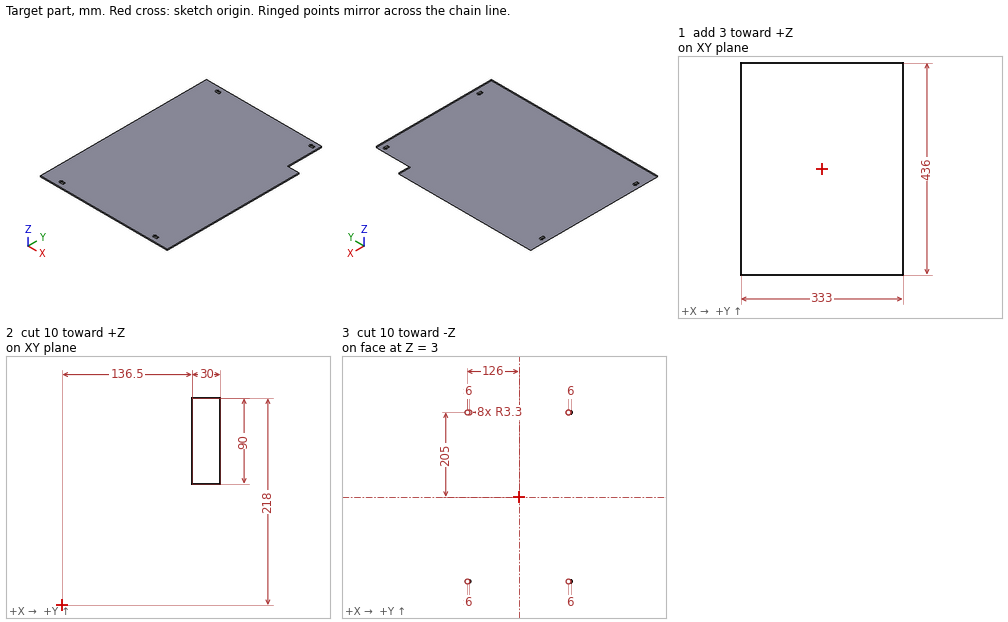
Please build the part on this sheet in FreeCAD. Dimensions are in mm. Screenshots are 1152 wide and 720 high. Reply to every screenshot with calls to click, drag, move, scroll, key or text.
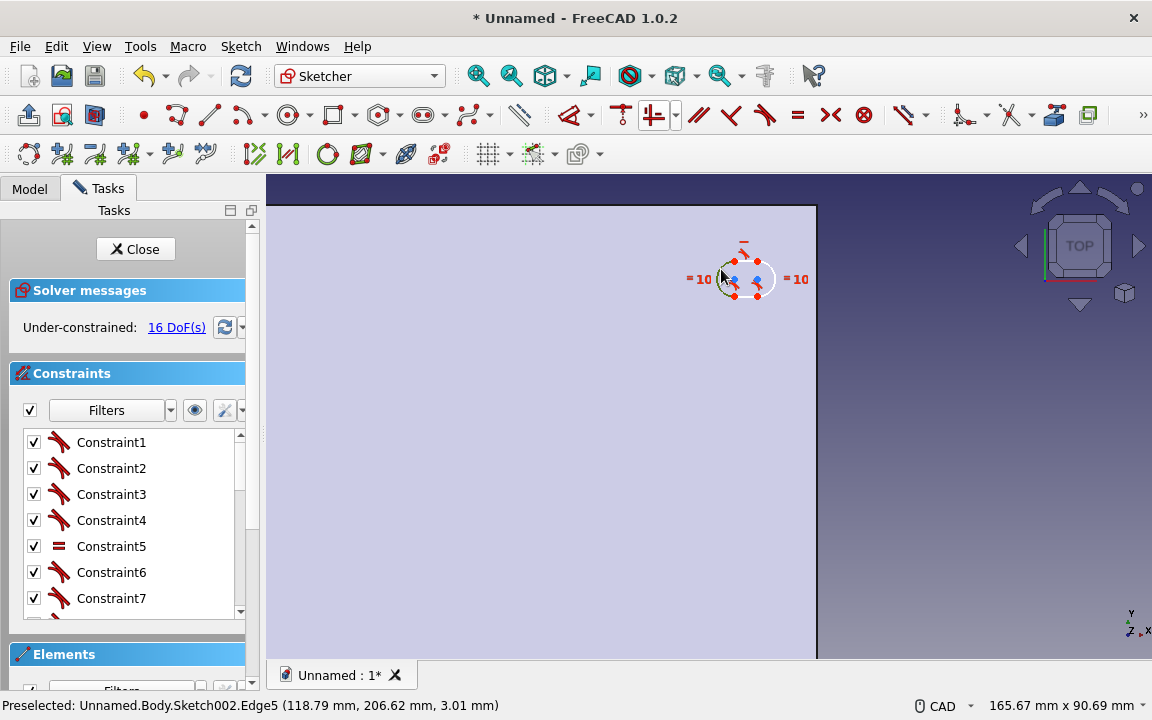
scroll(727, 267, down, 10)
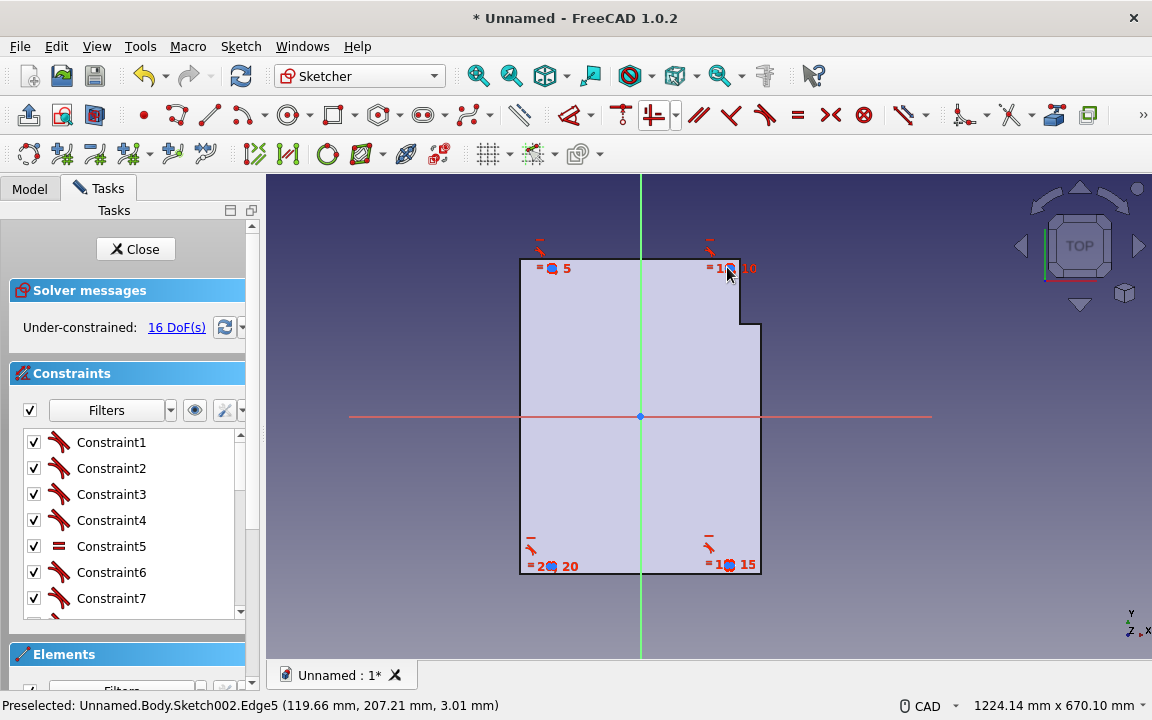
scroll(726, 564, up, 9)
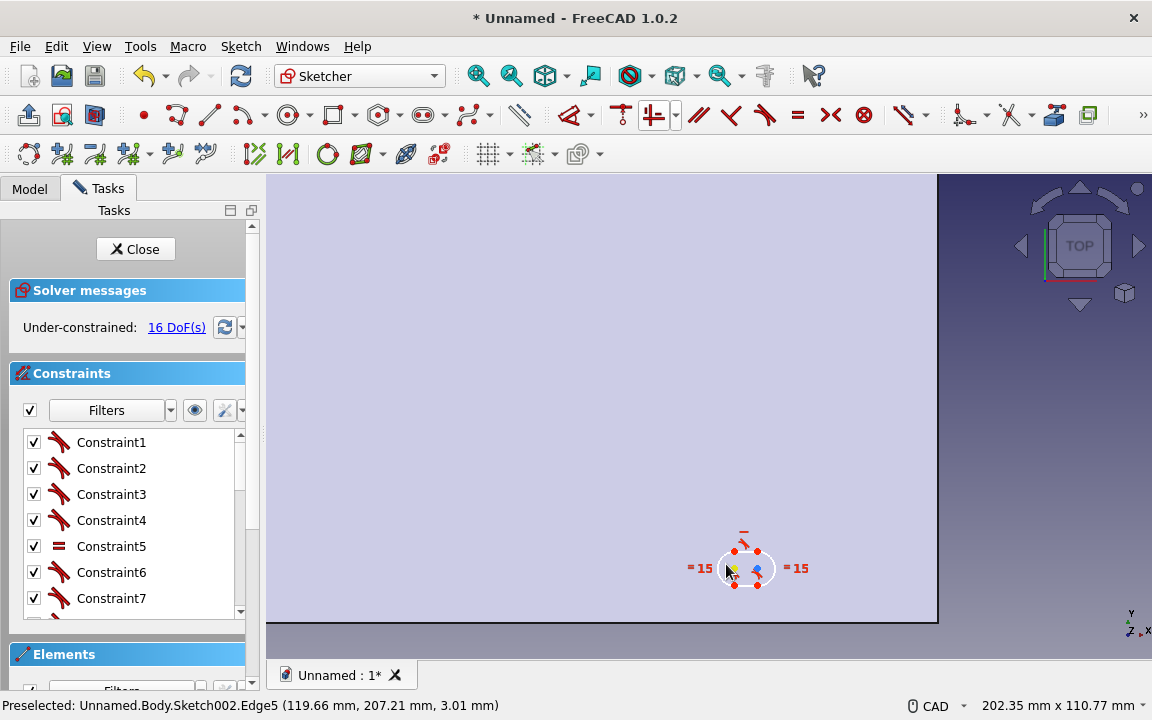
click(721, 559)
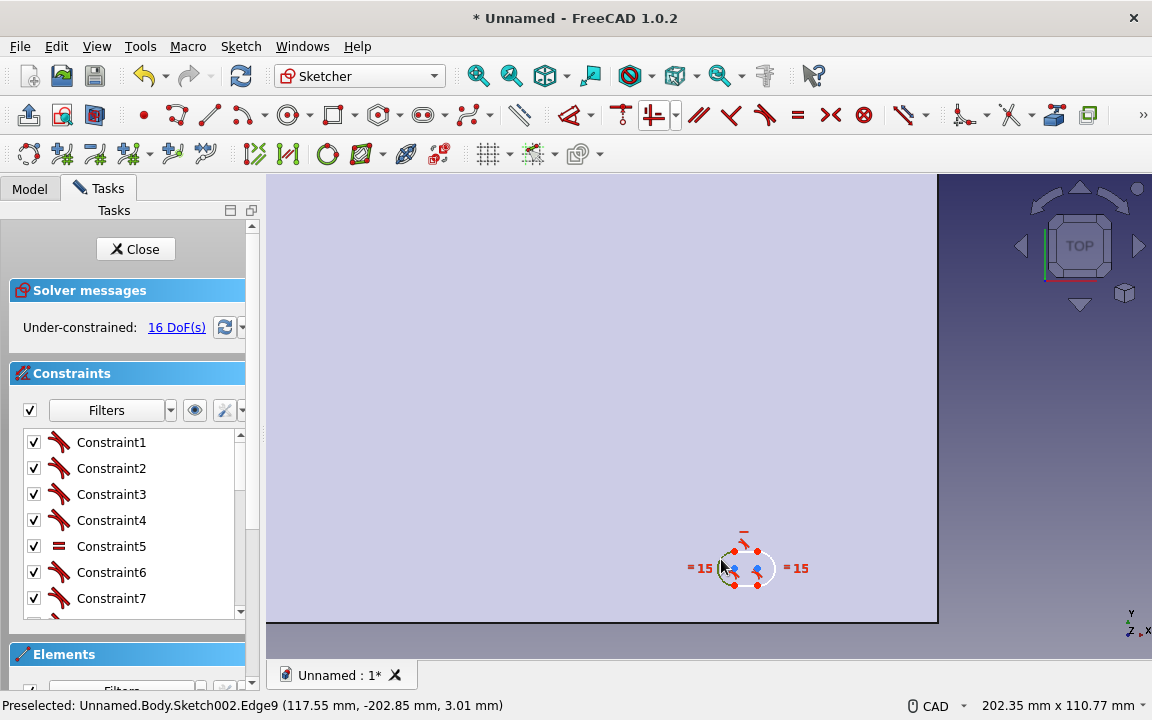
scroll(726, 565, down, 9)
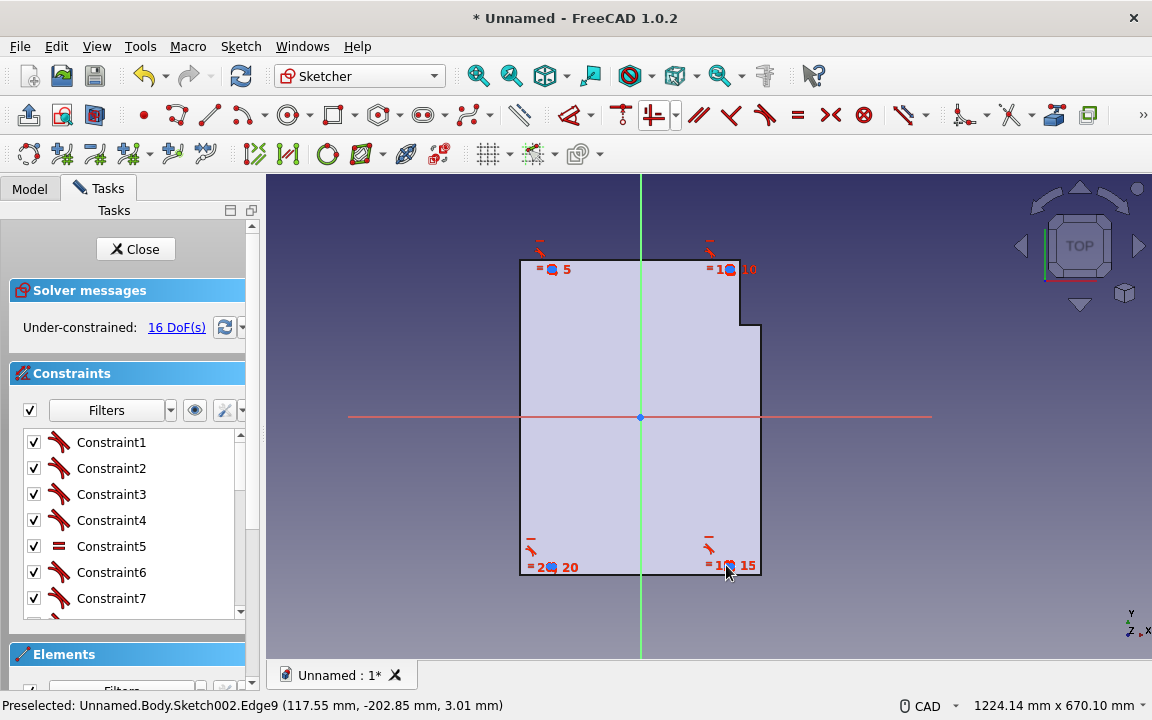
scroll(549, 567, up, 13)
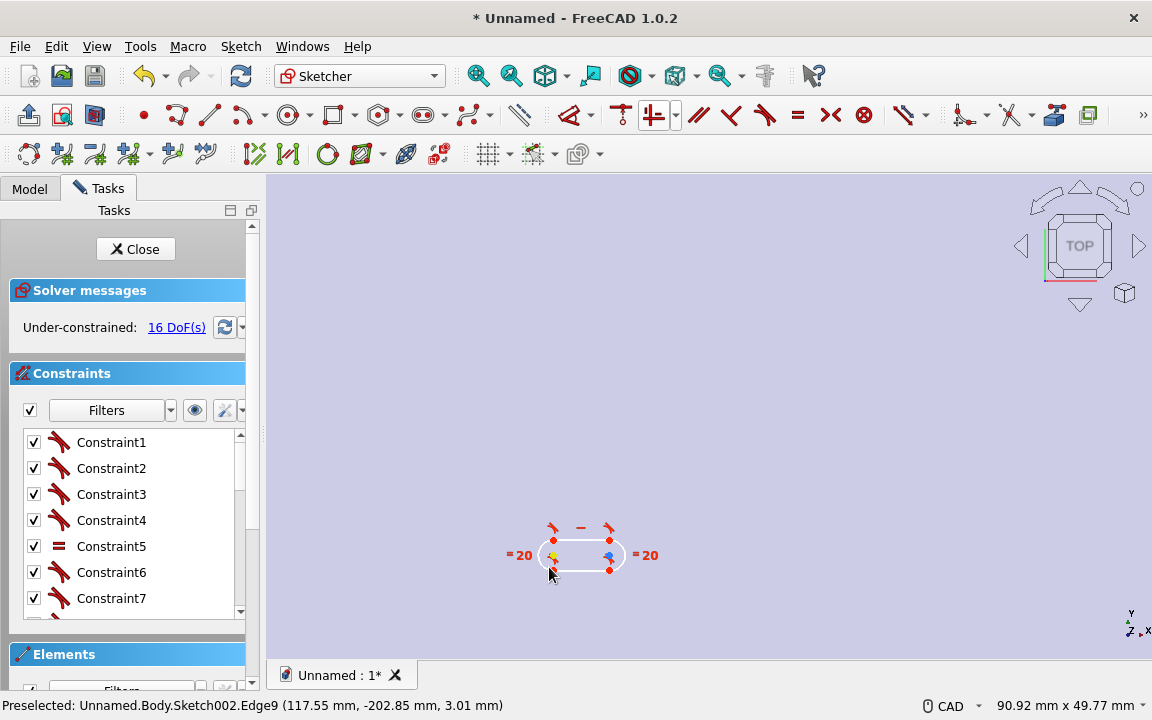
click(538, 555)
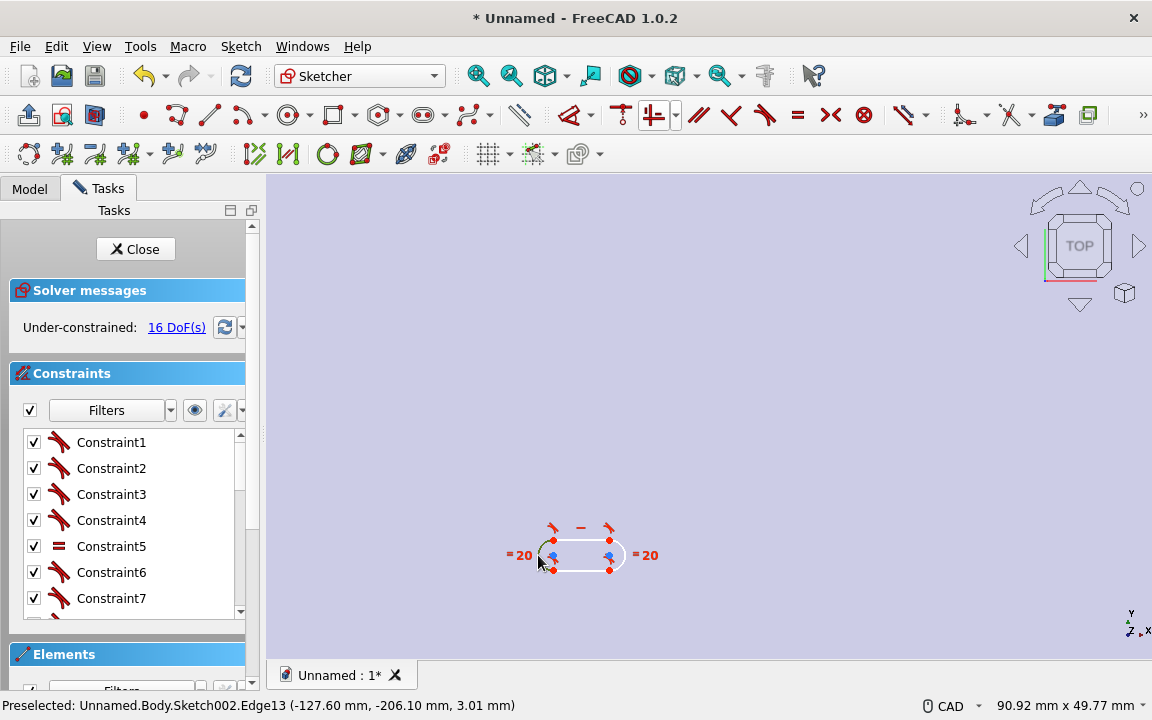
click(798, 116)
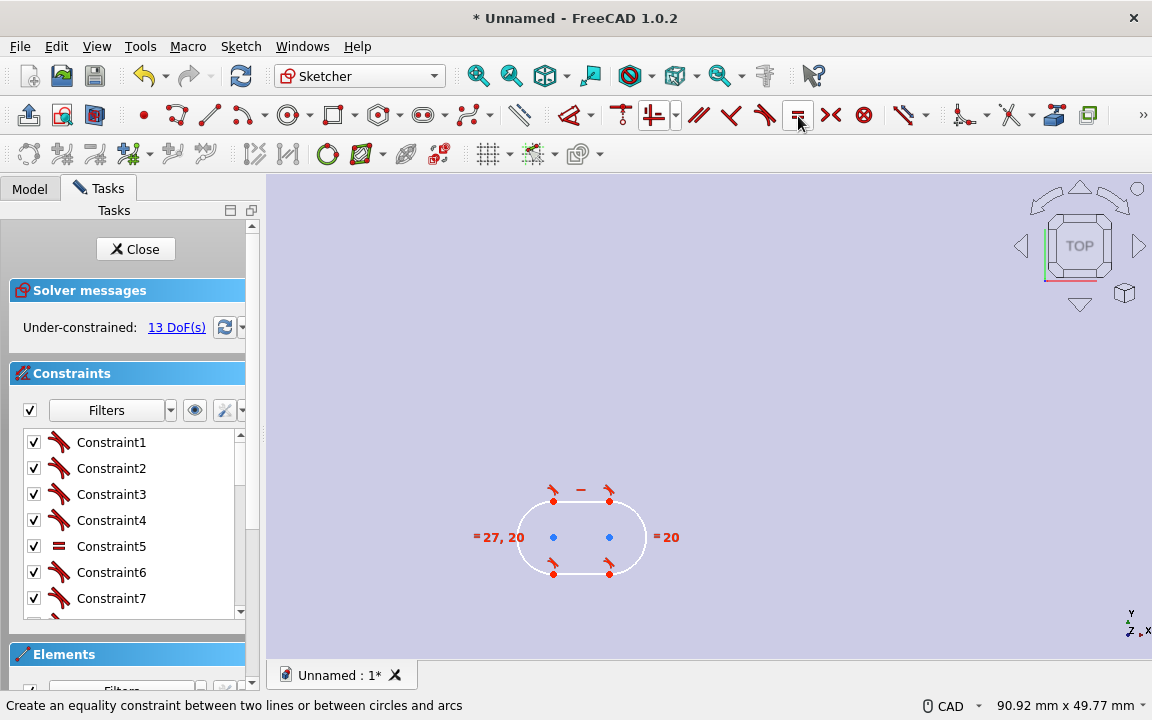
scroll(549, 567, down, 13)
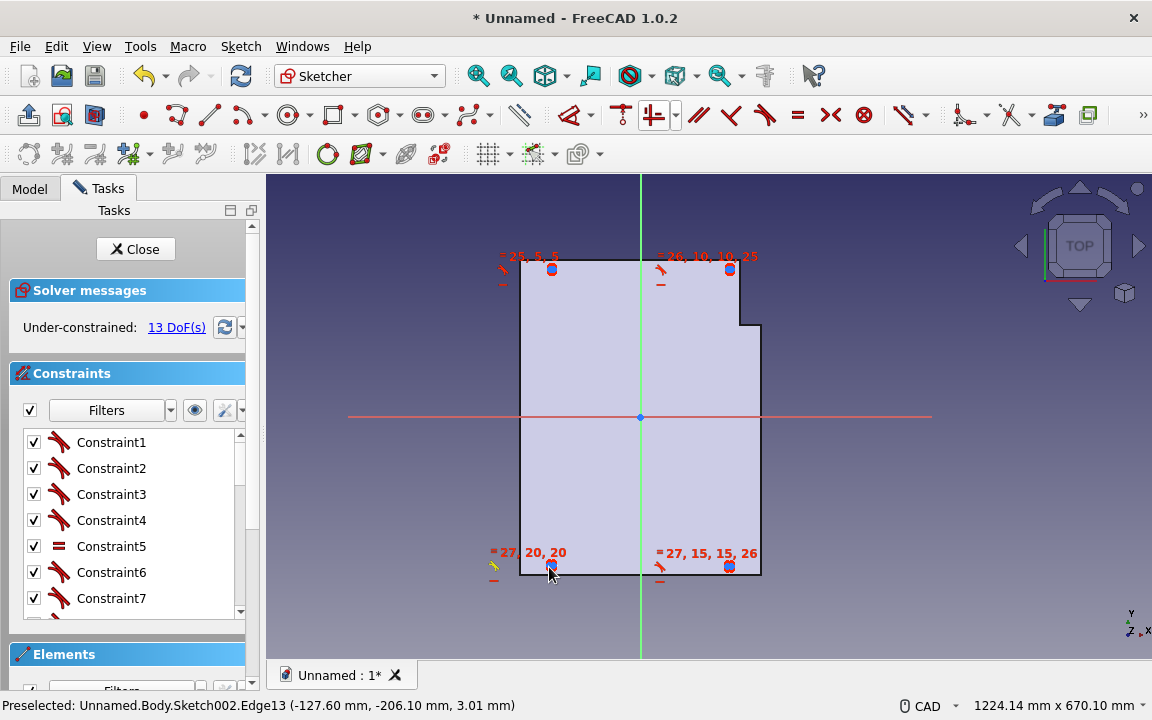
scroll(554, 270, up, 8)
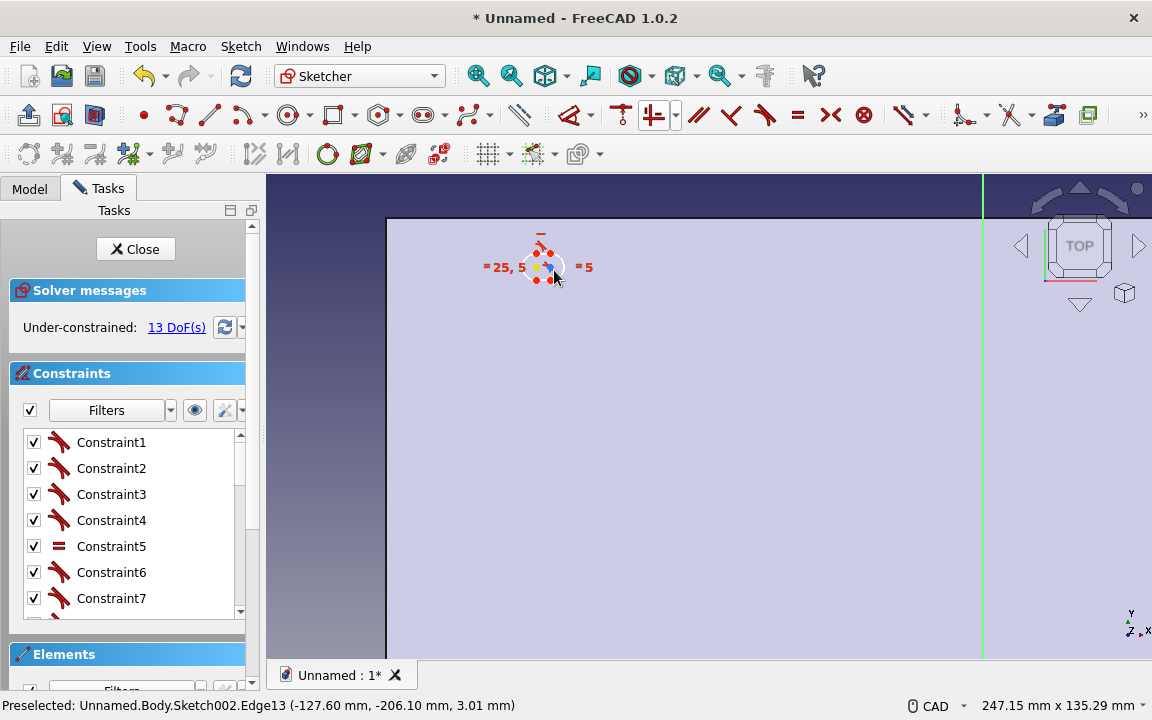
click(551, 267)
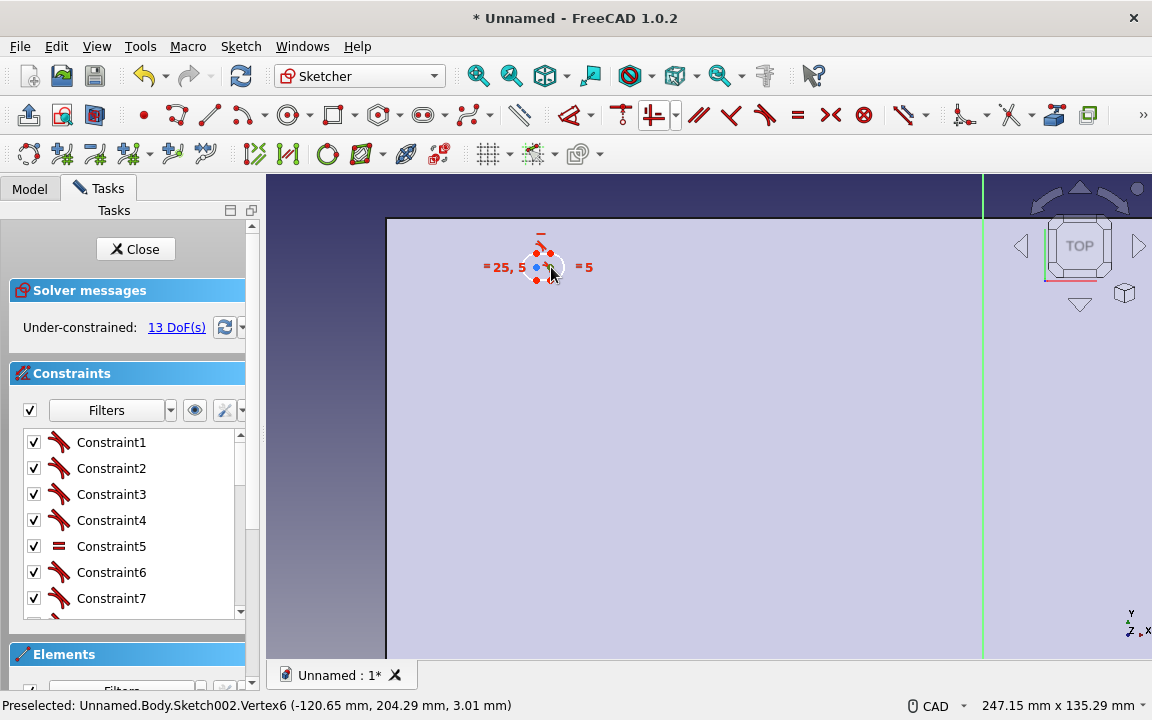
scroll(554, 269, down, 8)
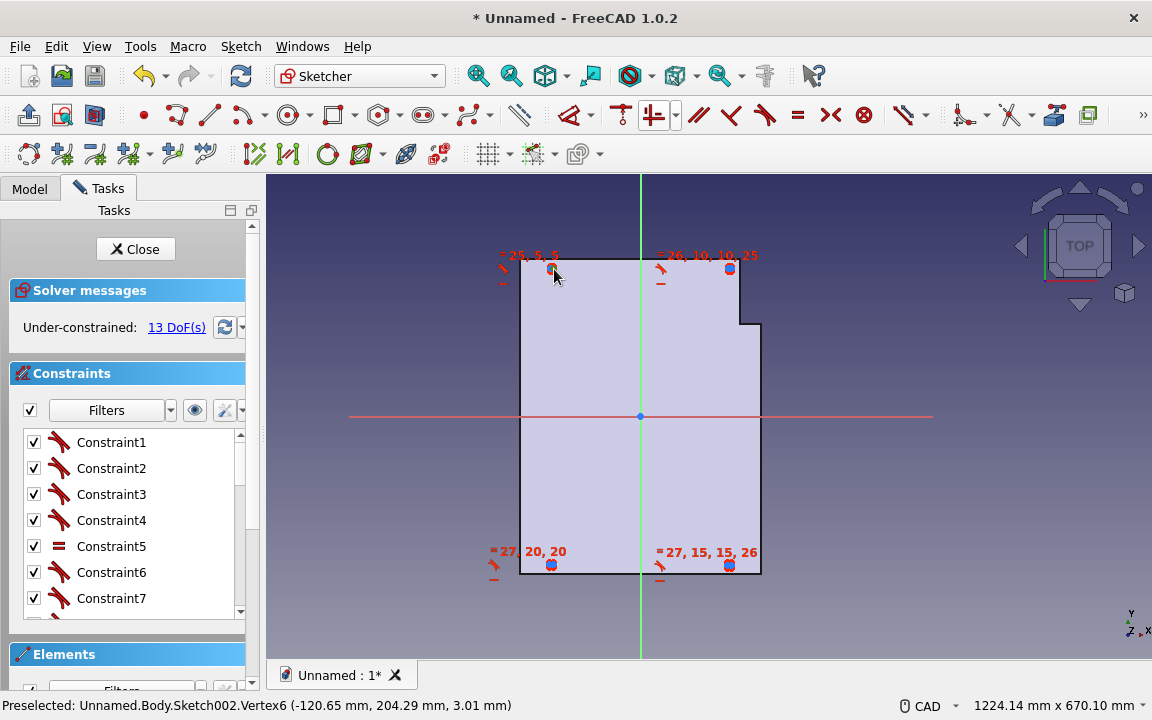
scroll(729, 269, up, 8)